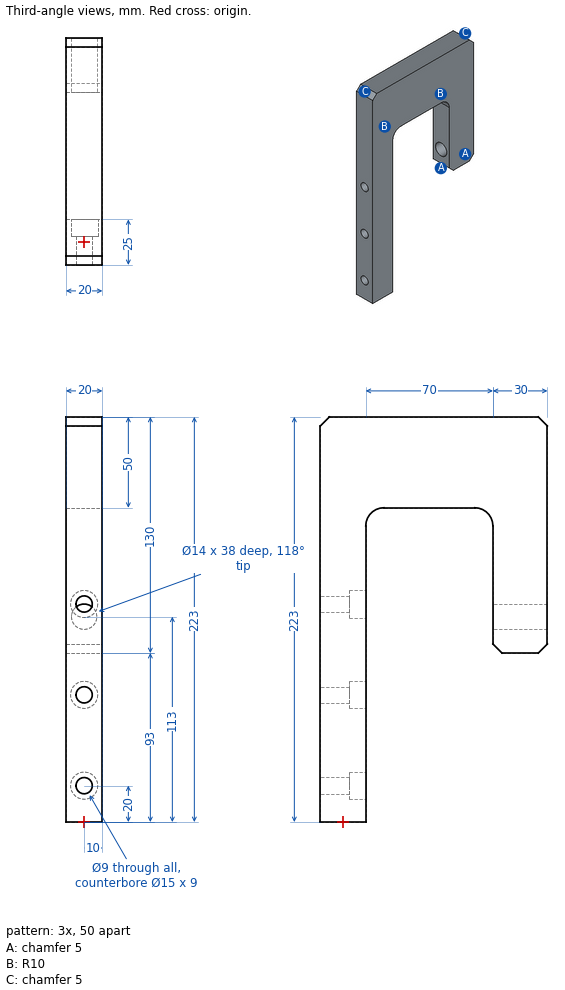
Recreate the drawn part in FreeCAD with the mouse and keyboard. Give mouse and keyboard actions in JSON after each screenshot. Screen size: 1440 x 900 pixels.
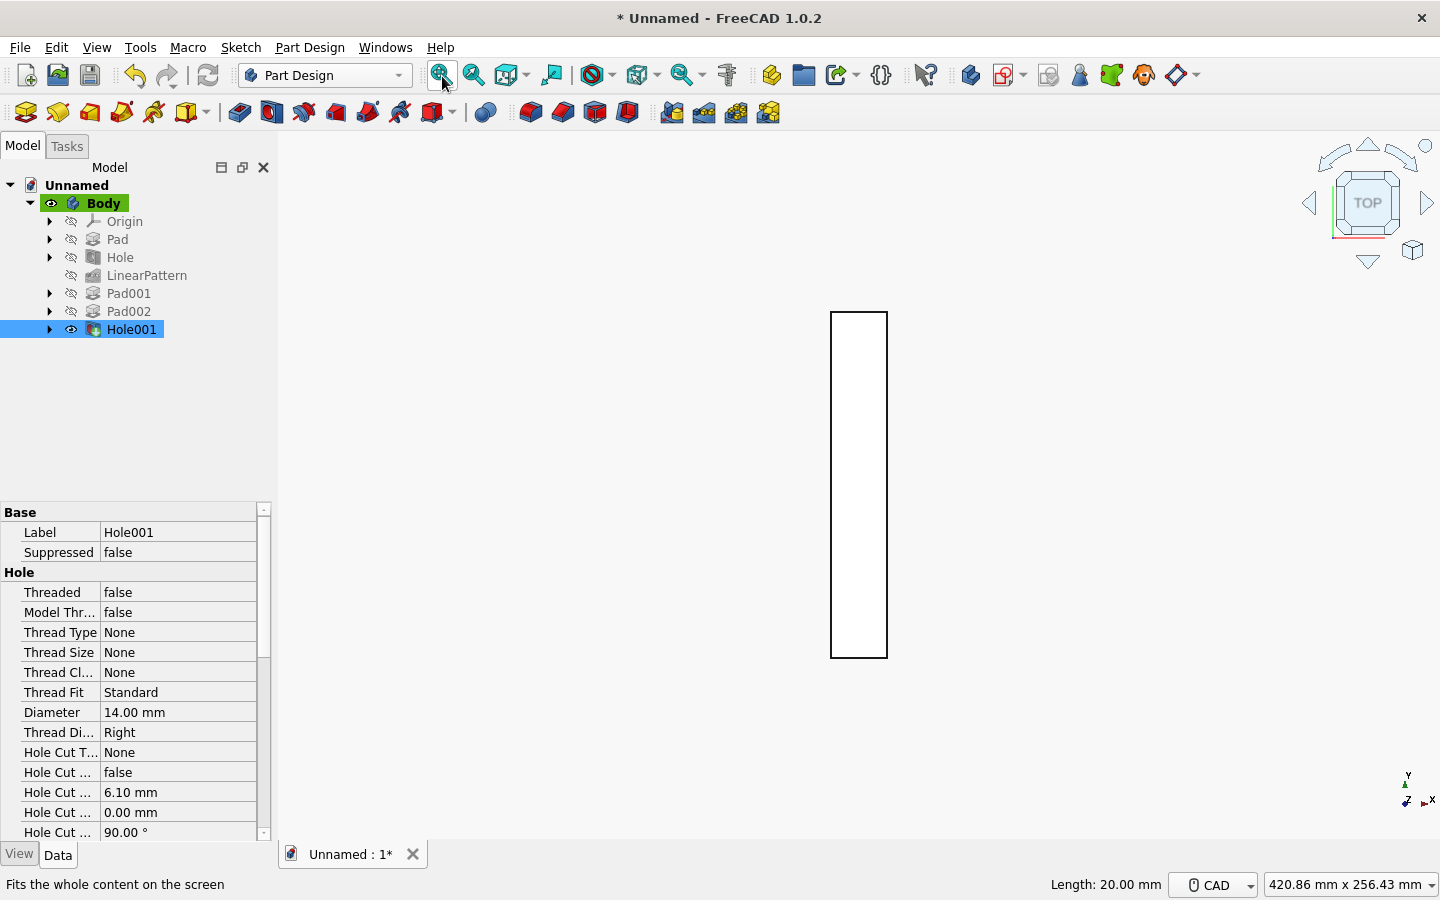
{"action": "key", "text": "1"}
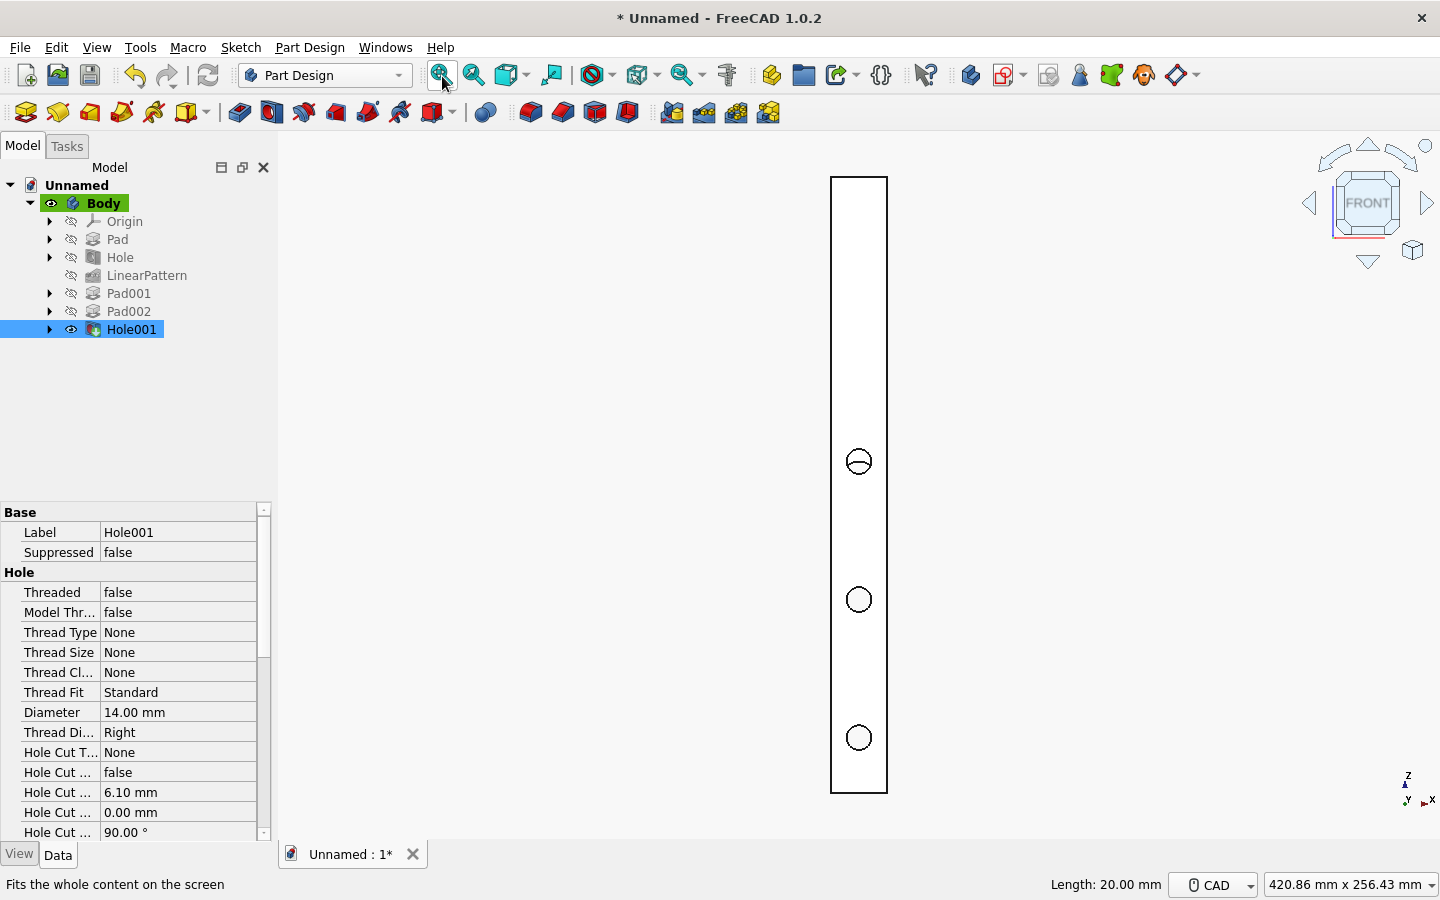
{"action": "key", "text": "3"}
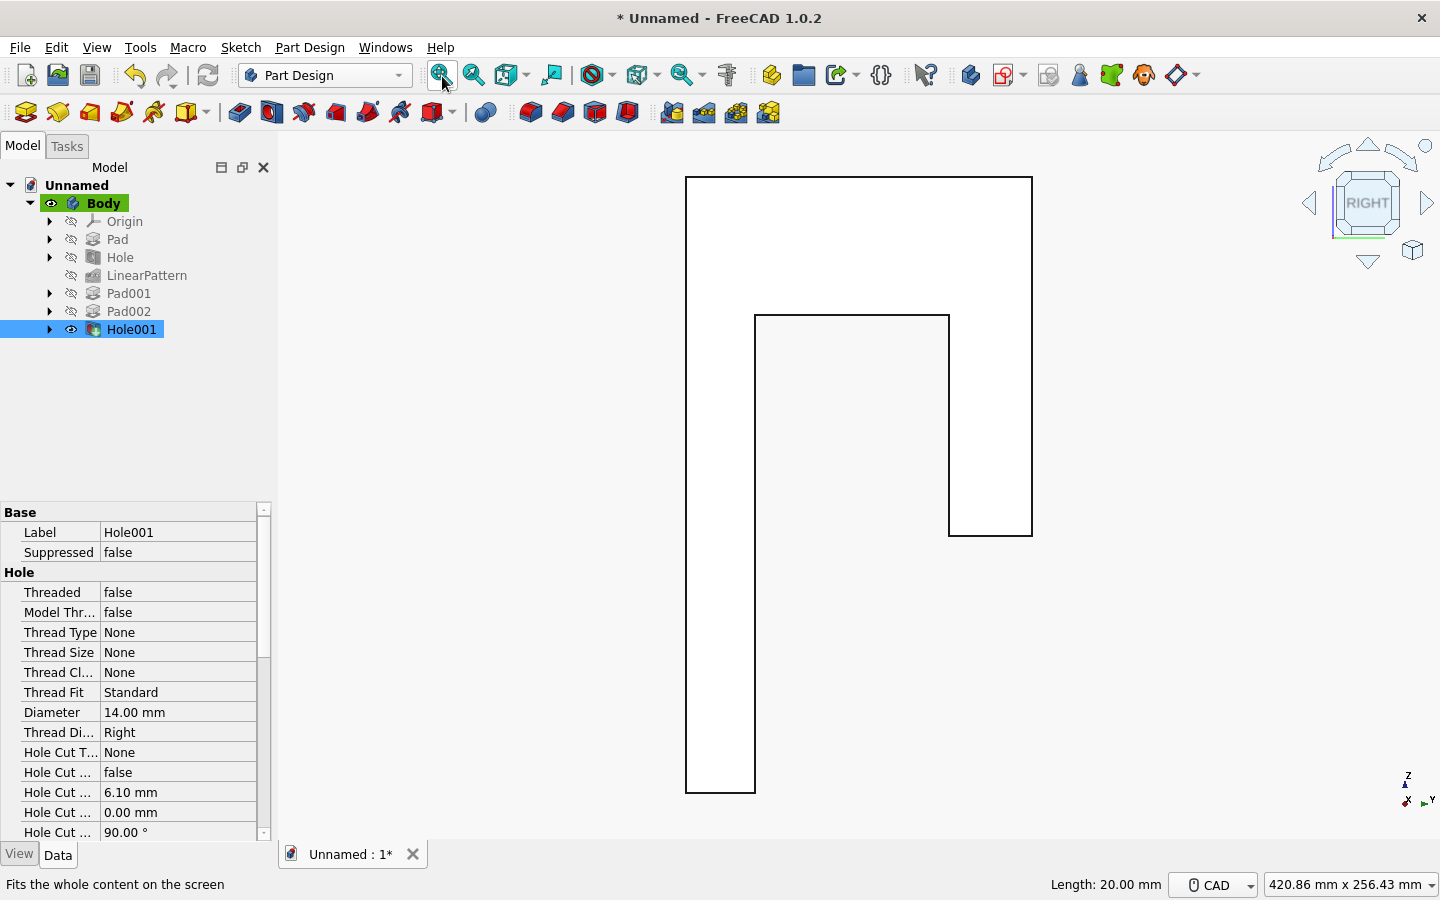
{"action": "key", "text": "5"}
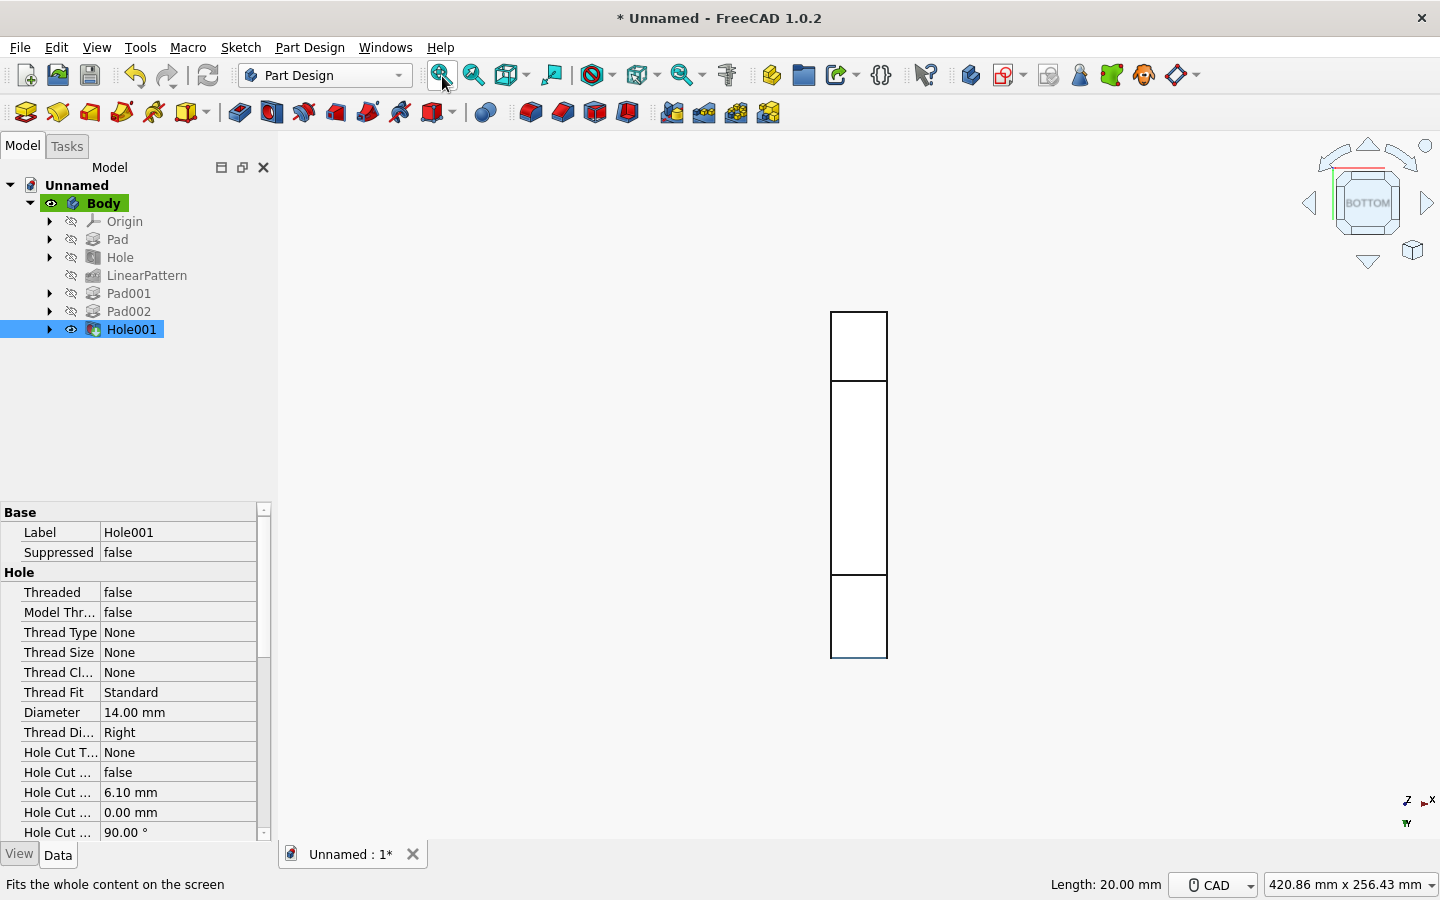
{"action": "left_click", "coordinate": [859, 574], "text": "ctrl"}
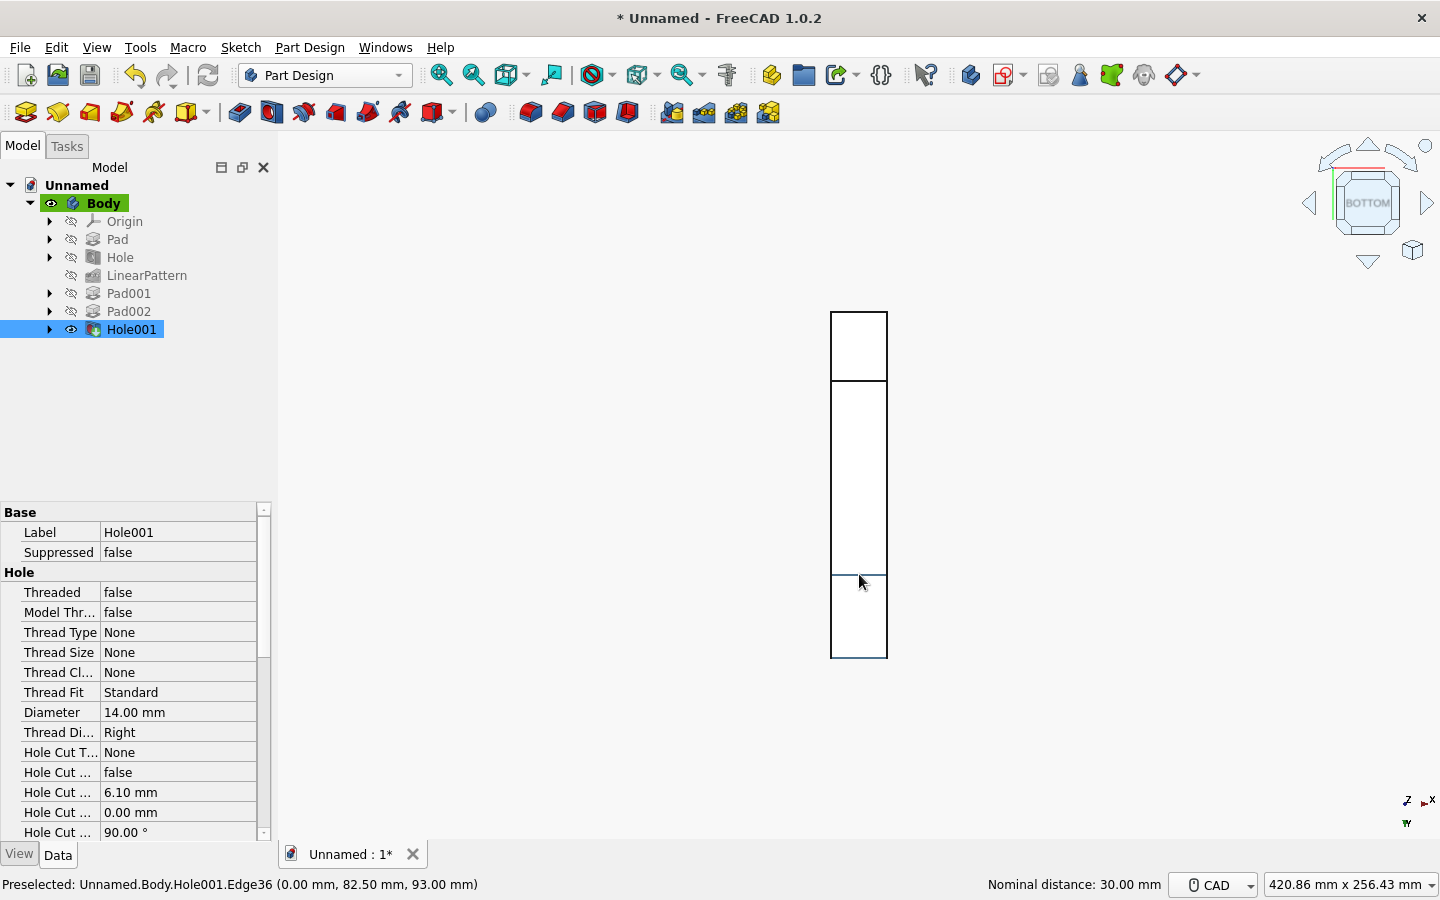
{"action": "left_click", "coordinate": [564, 112]}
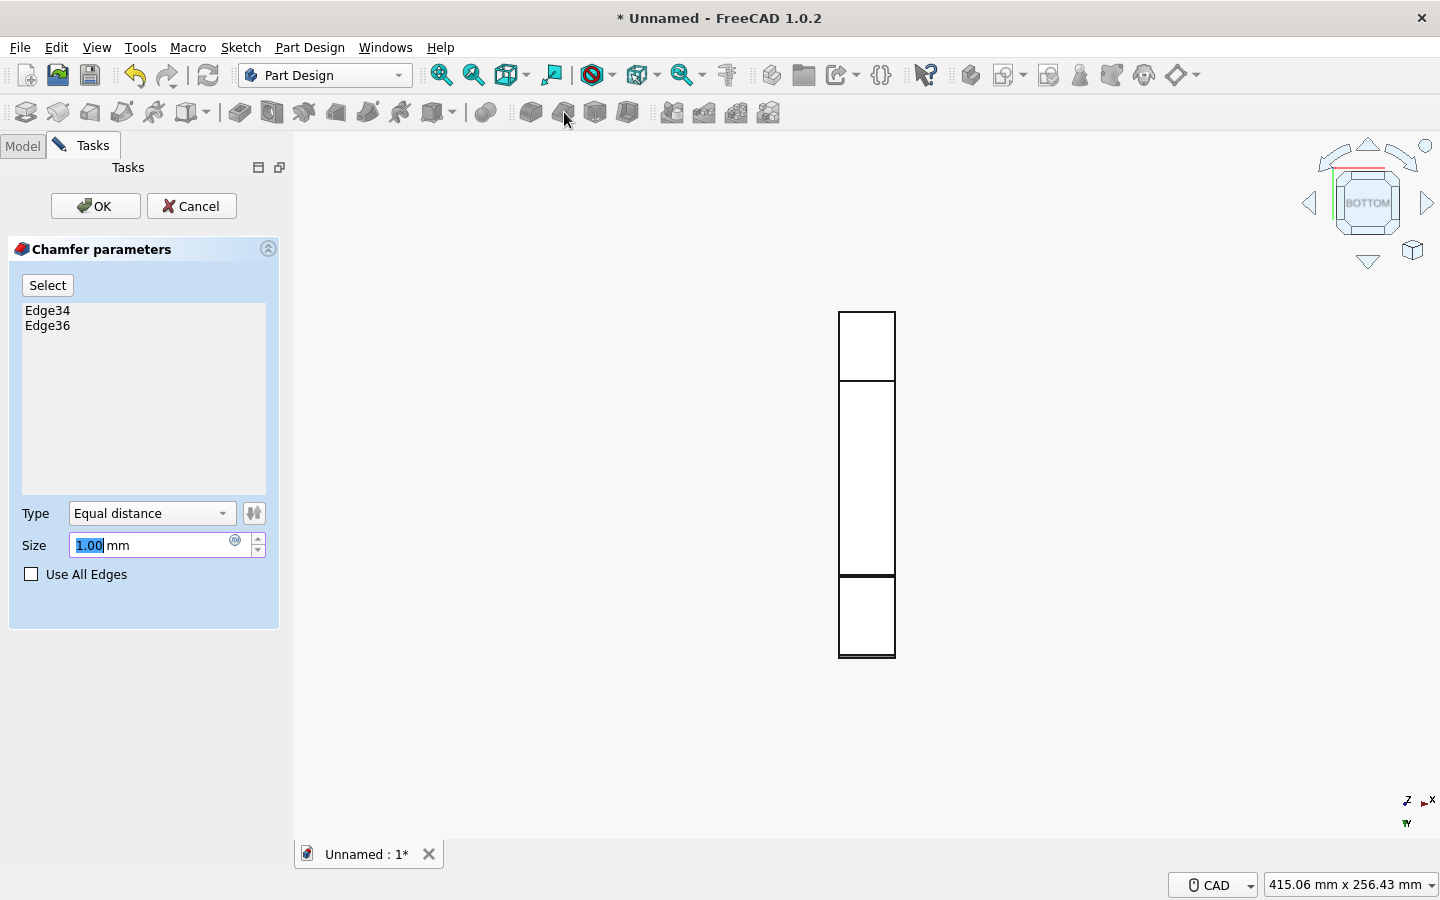
{"action": "type", "text": "5"}
{"action": "key", "text": "Tab"}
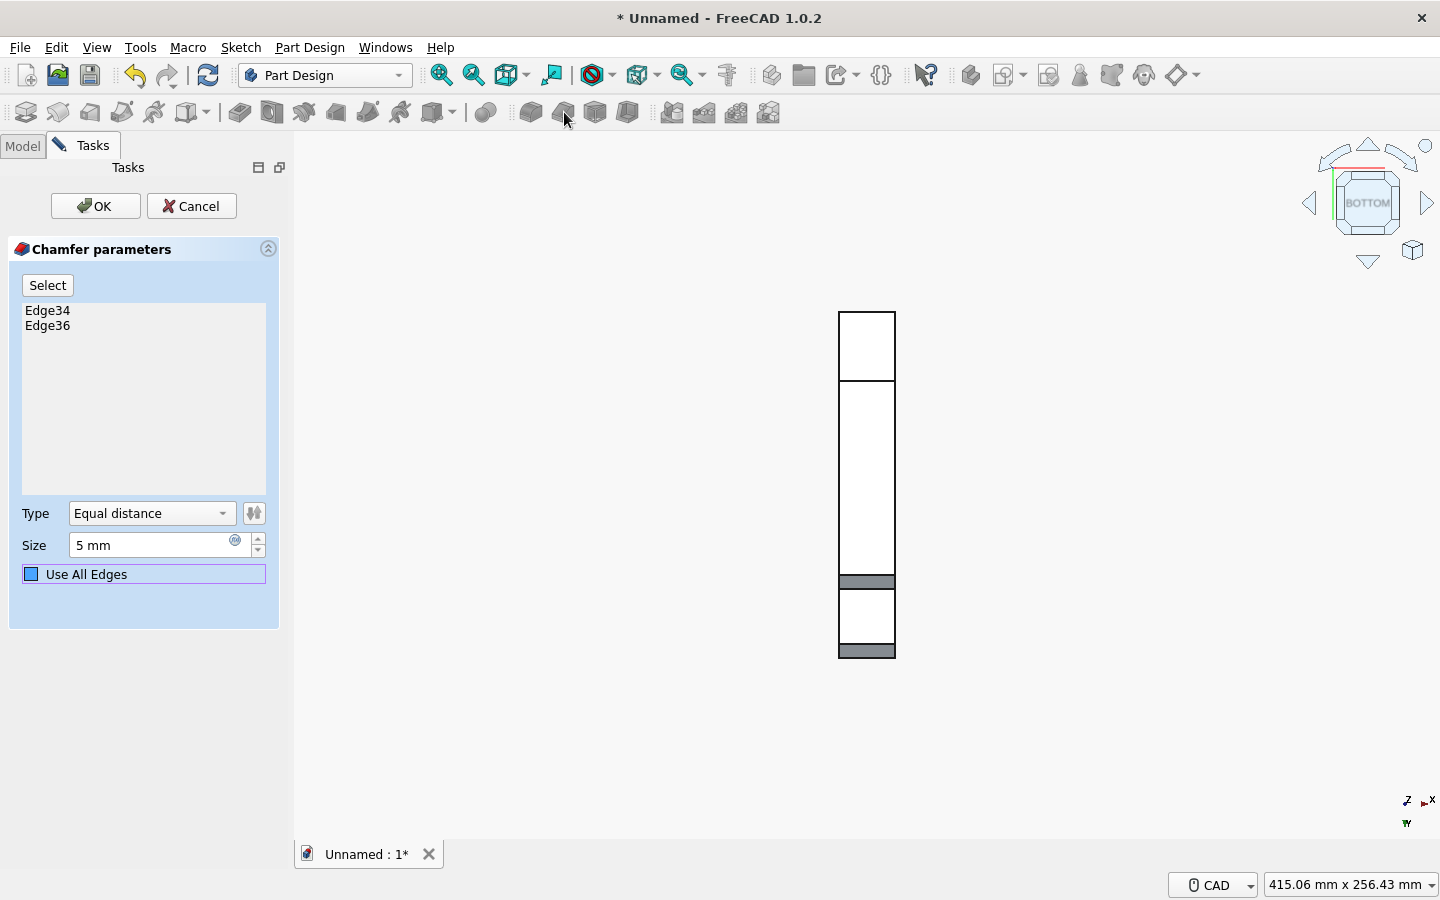
{"action": "left_click", "coordinate": [96, 206]}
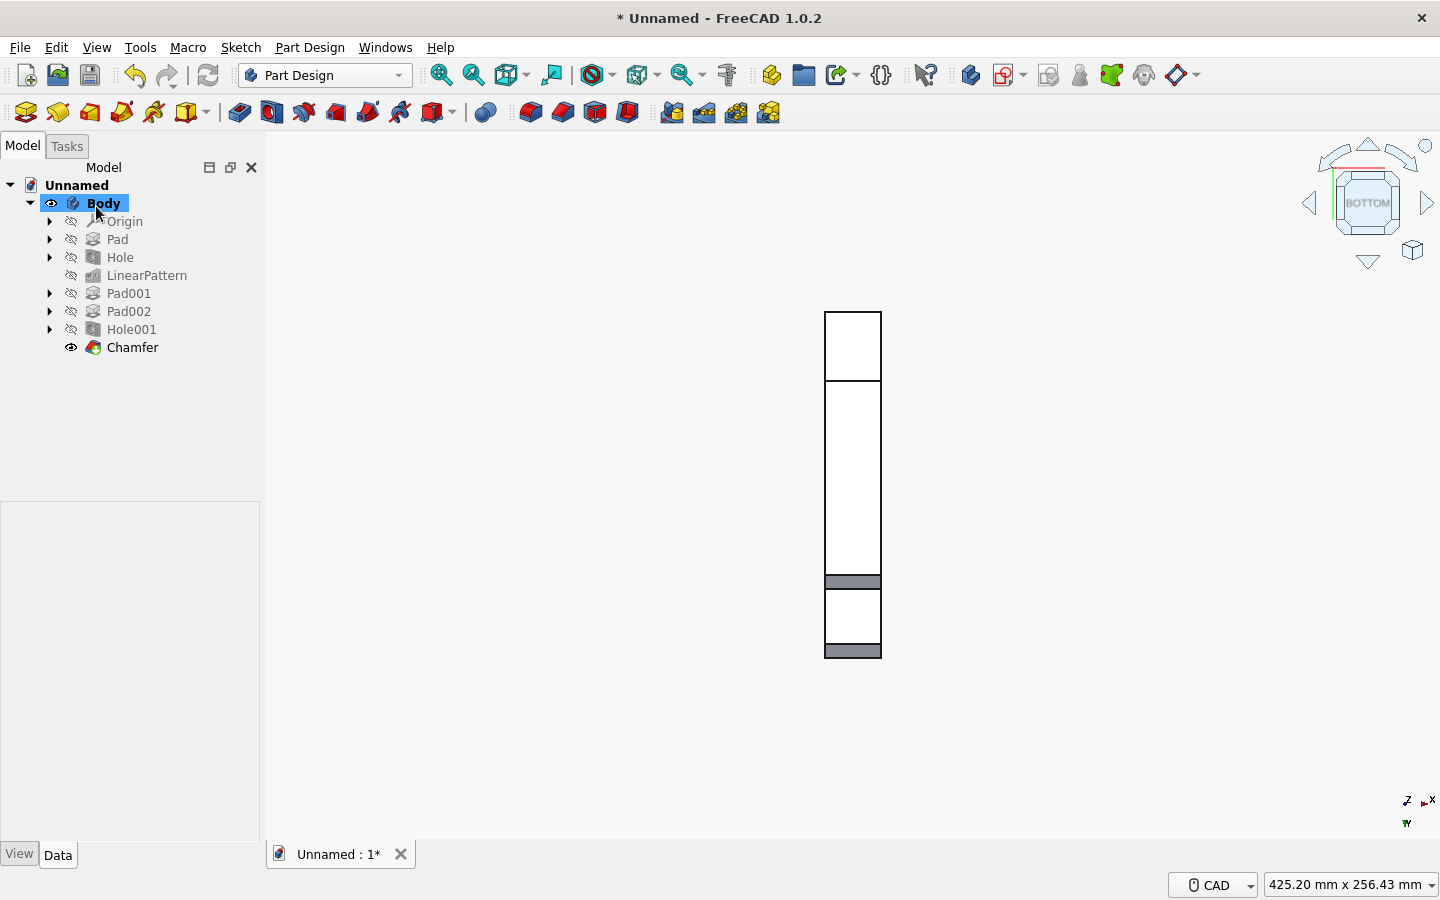
{"action": "key", "text": "0"}